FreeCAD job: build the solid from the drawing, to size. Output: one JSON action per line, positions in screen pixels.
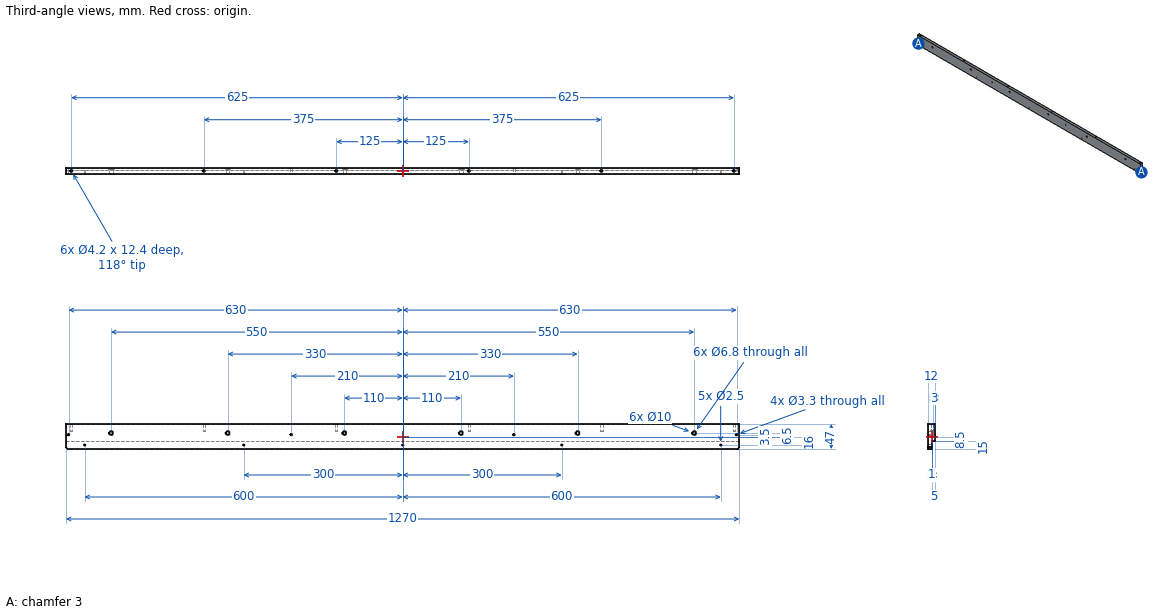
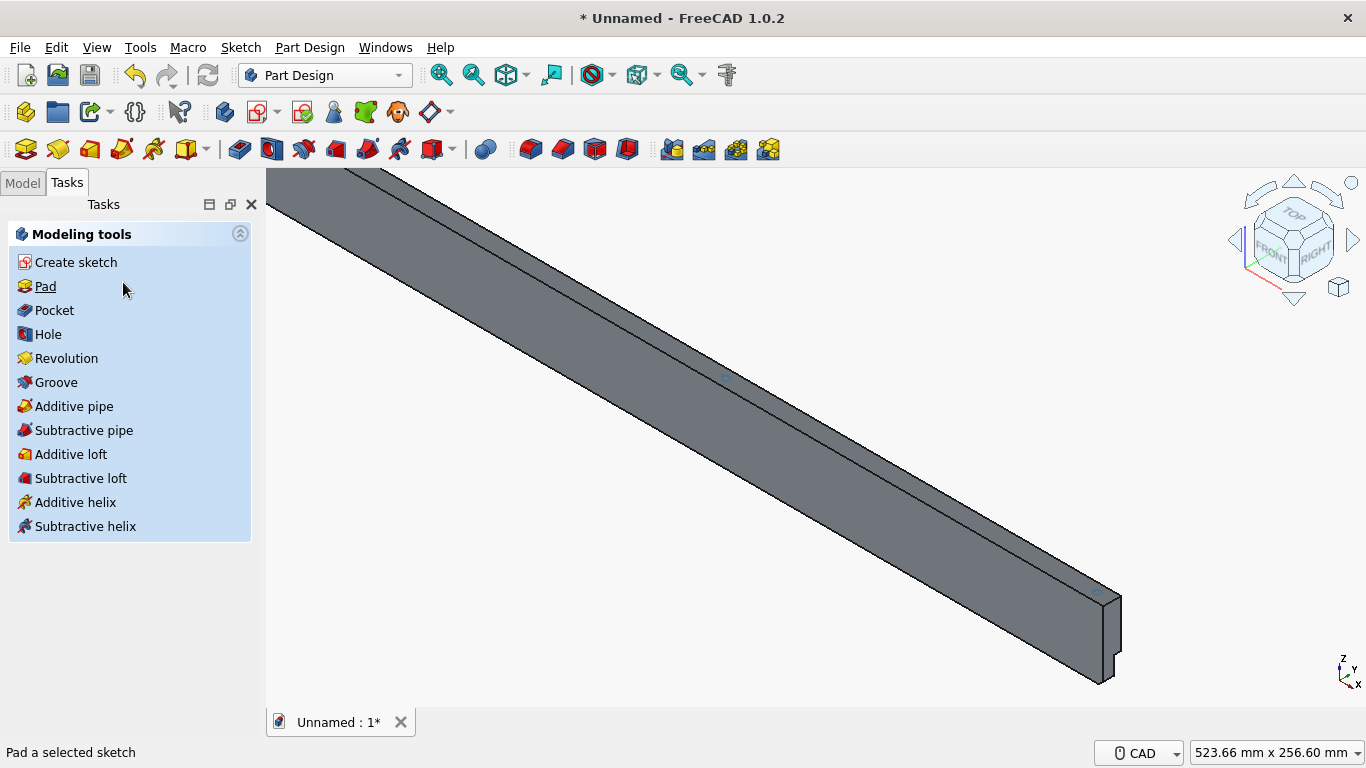
{"action": "left_click", "coordinate": [272, 150]}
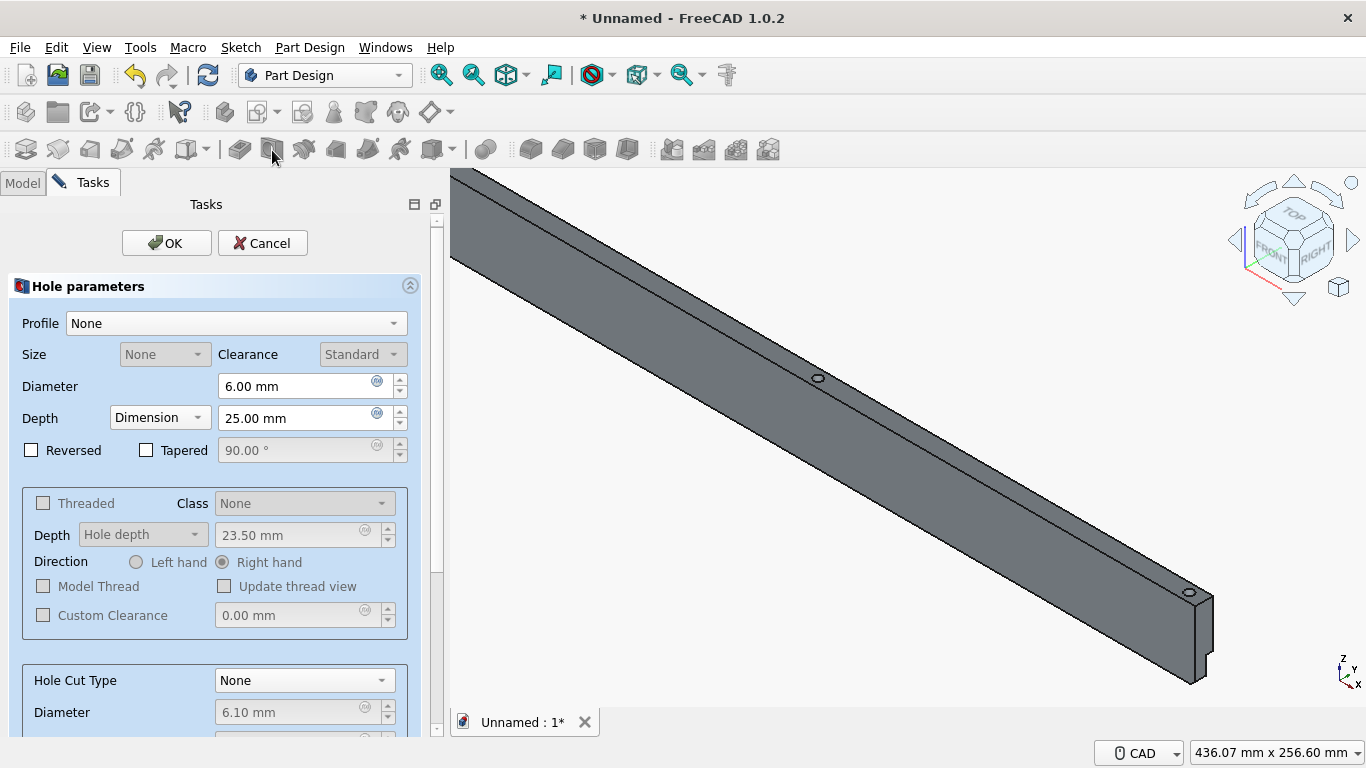
{"action": "triple_click", "coordinate": [305, 386]}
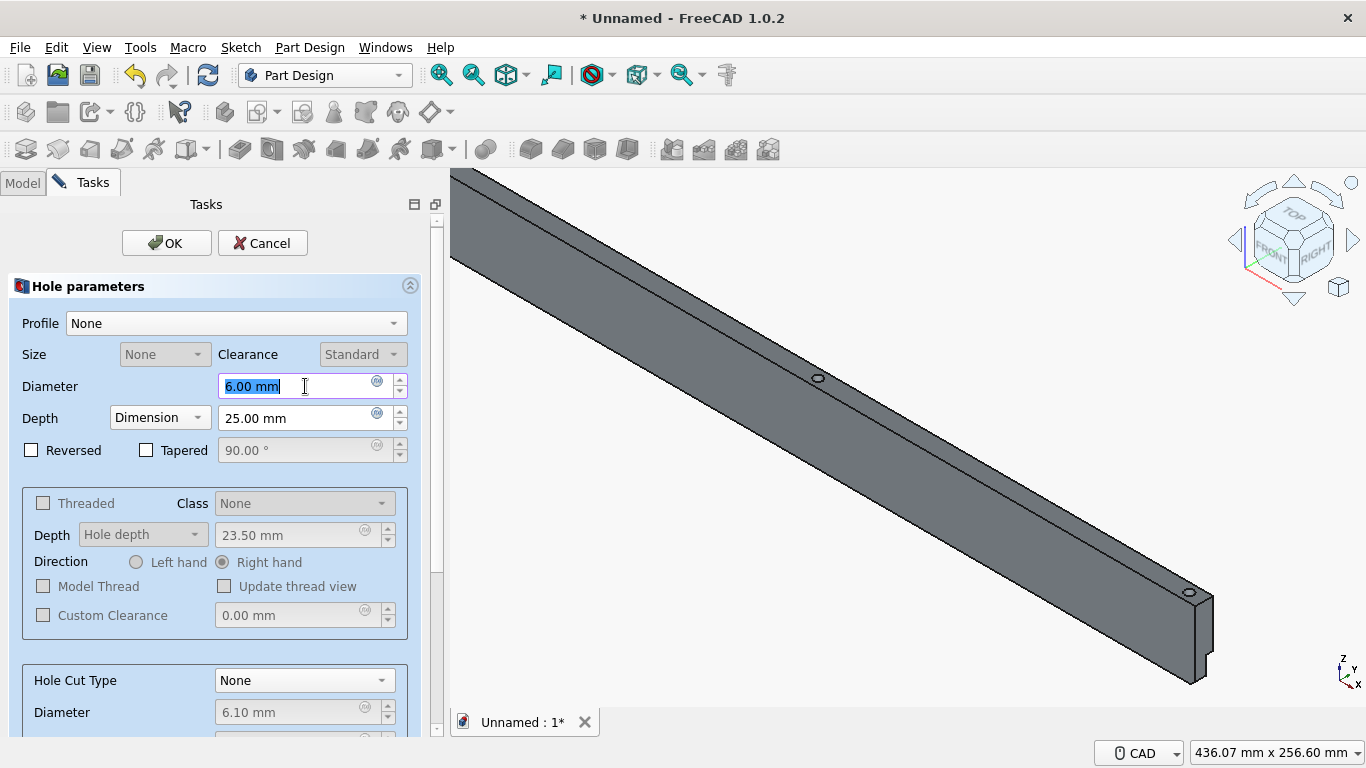
{"action": "type", "text": "4.2"}
{"action": "key", "text": "Tab"}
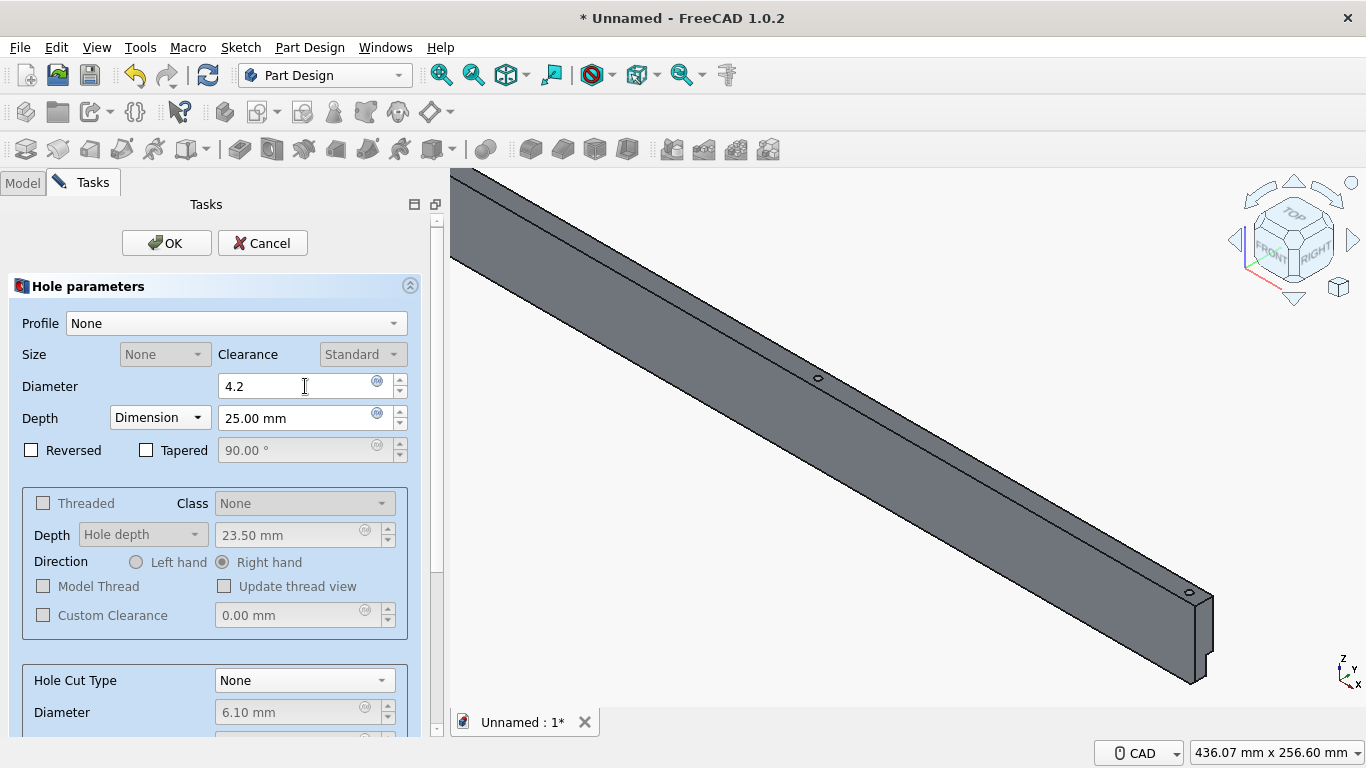
{"action": "triple_click", "coordinate": [305, 418]}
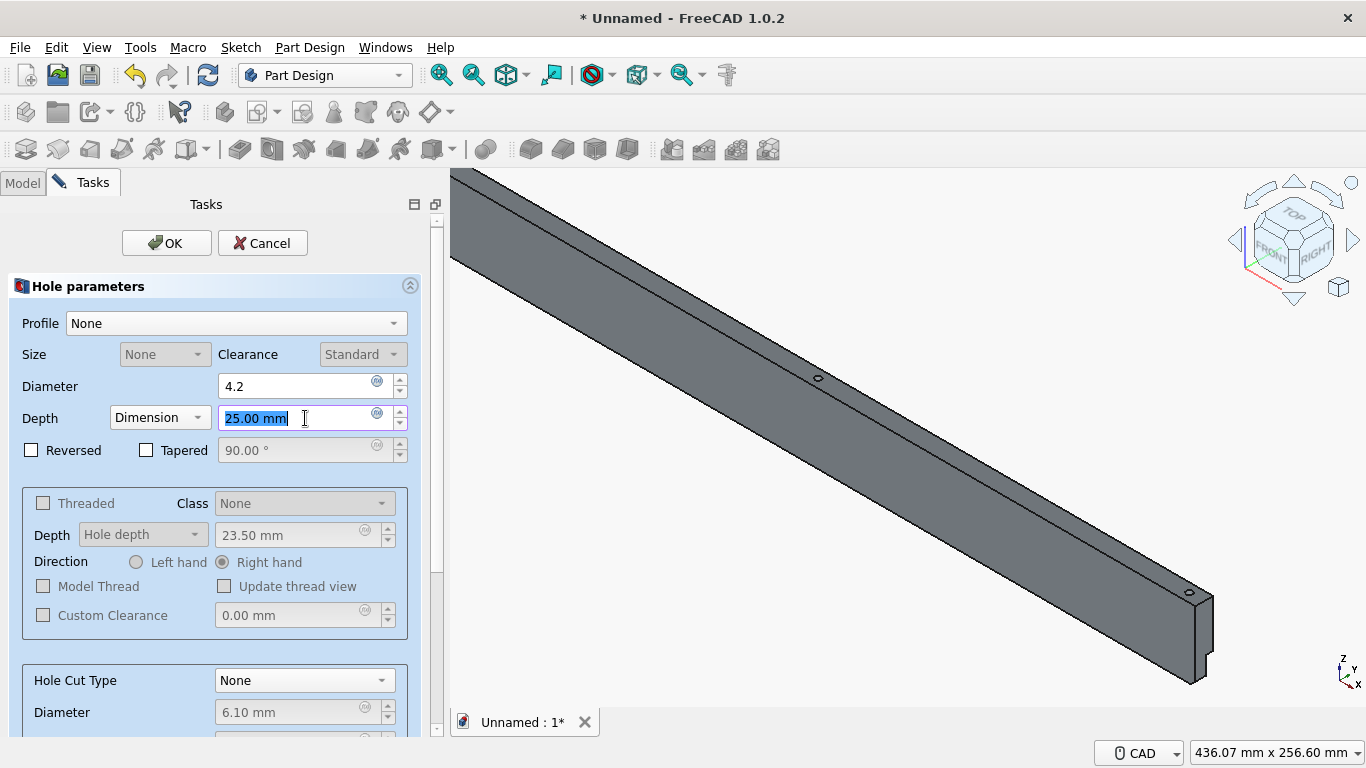
{"action": "type", "text": "12.4"}
{"action": "key", "text": "Tab"}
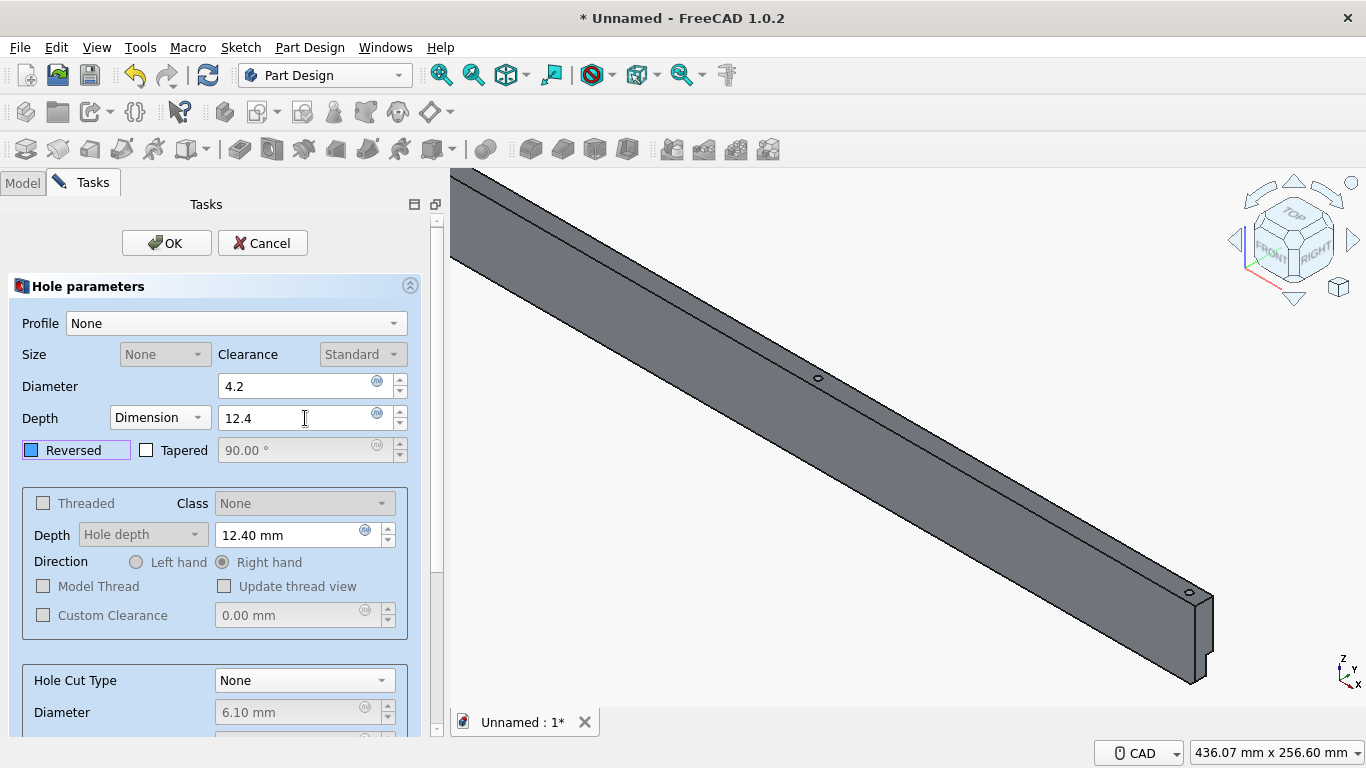
{"action": "left_click", "coordinate": [167, 243]}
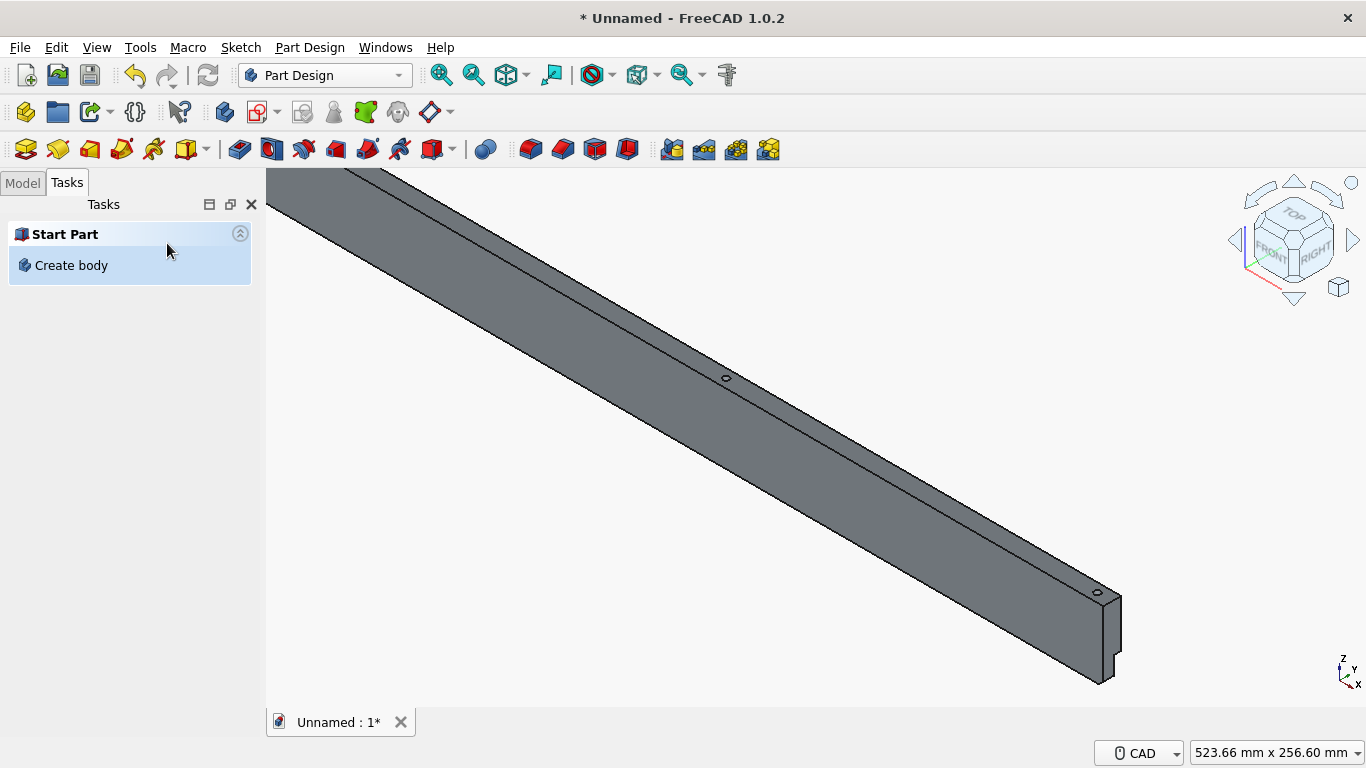
{"action": "left_click", "coordinate": [442, 76]}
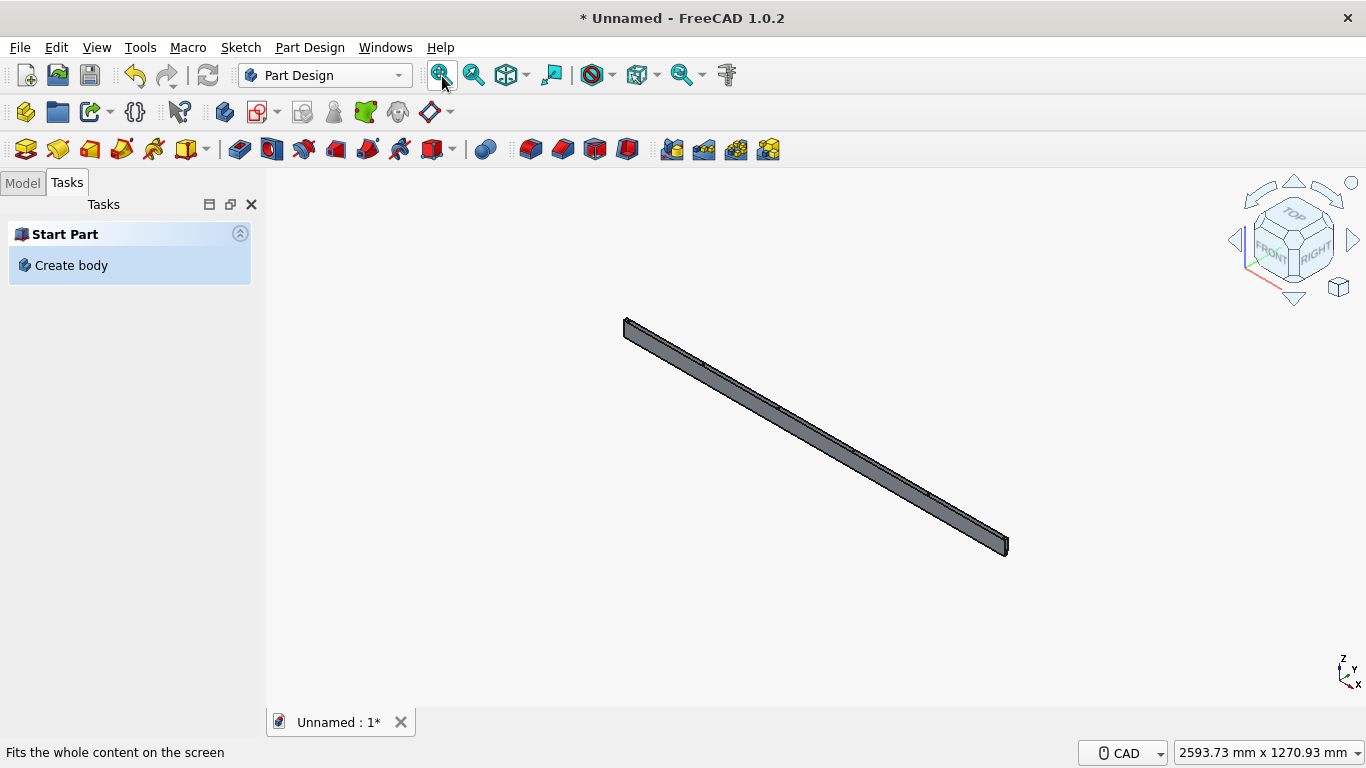
{"action": "key", "text": "4"}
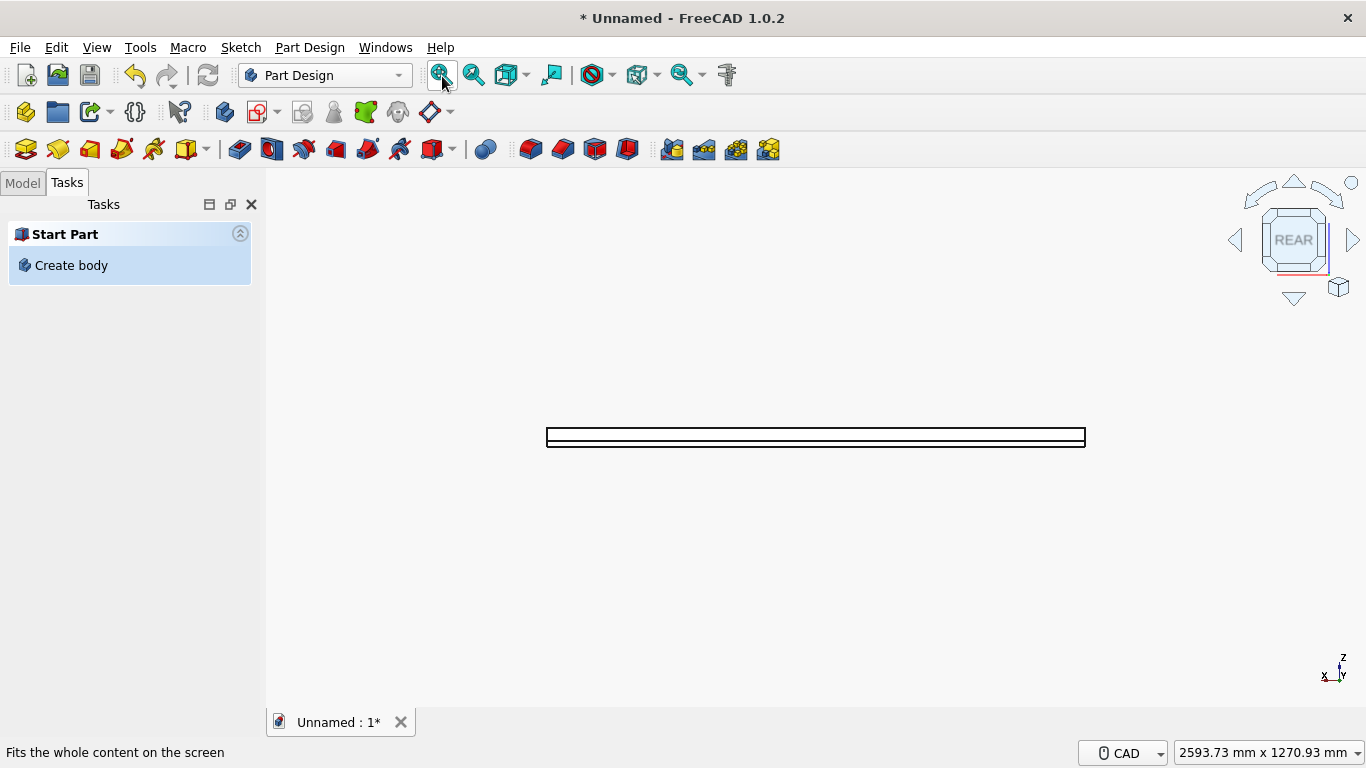
{"action": "left_click", "coordinate": [585, 431]}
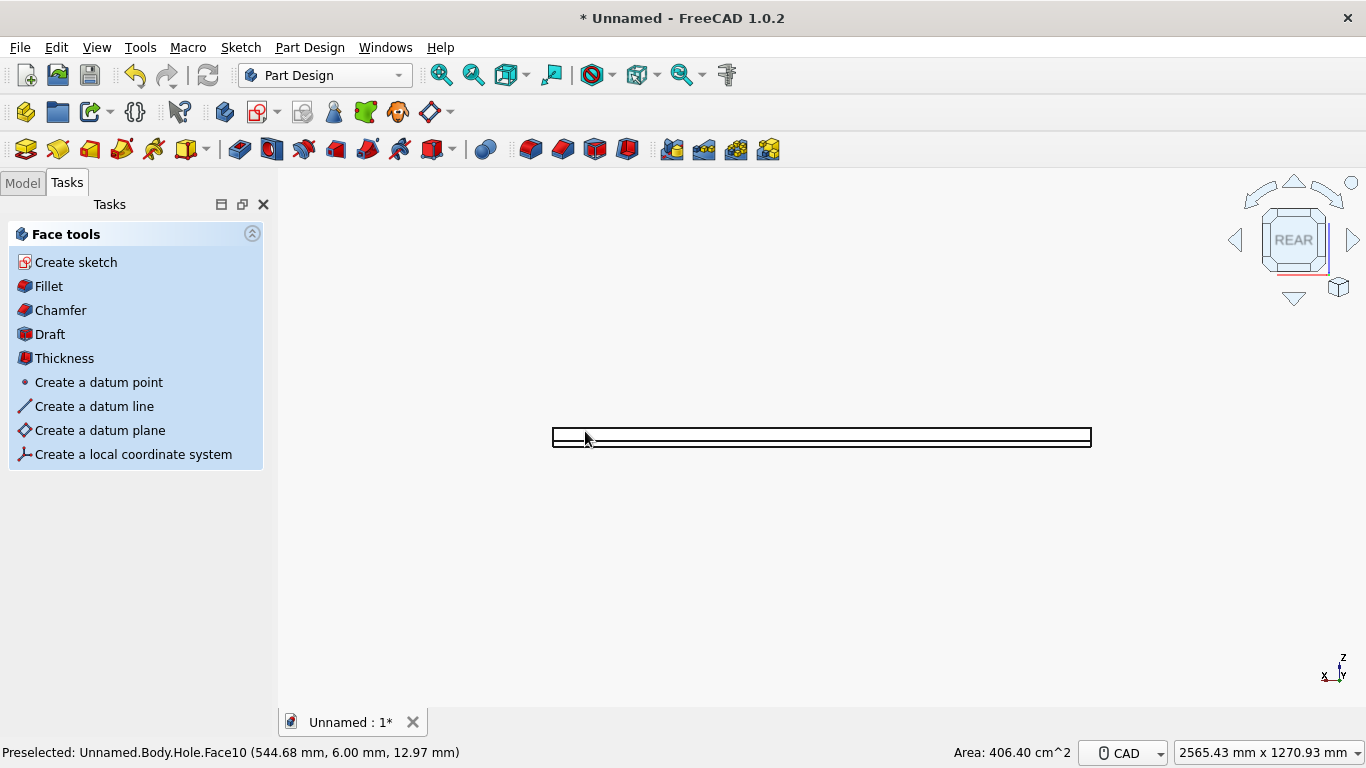
{"action": "left_click", "coordinate": [258, 112]}